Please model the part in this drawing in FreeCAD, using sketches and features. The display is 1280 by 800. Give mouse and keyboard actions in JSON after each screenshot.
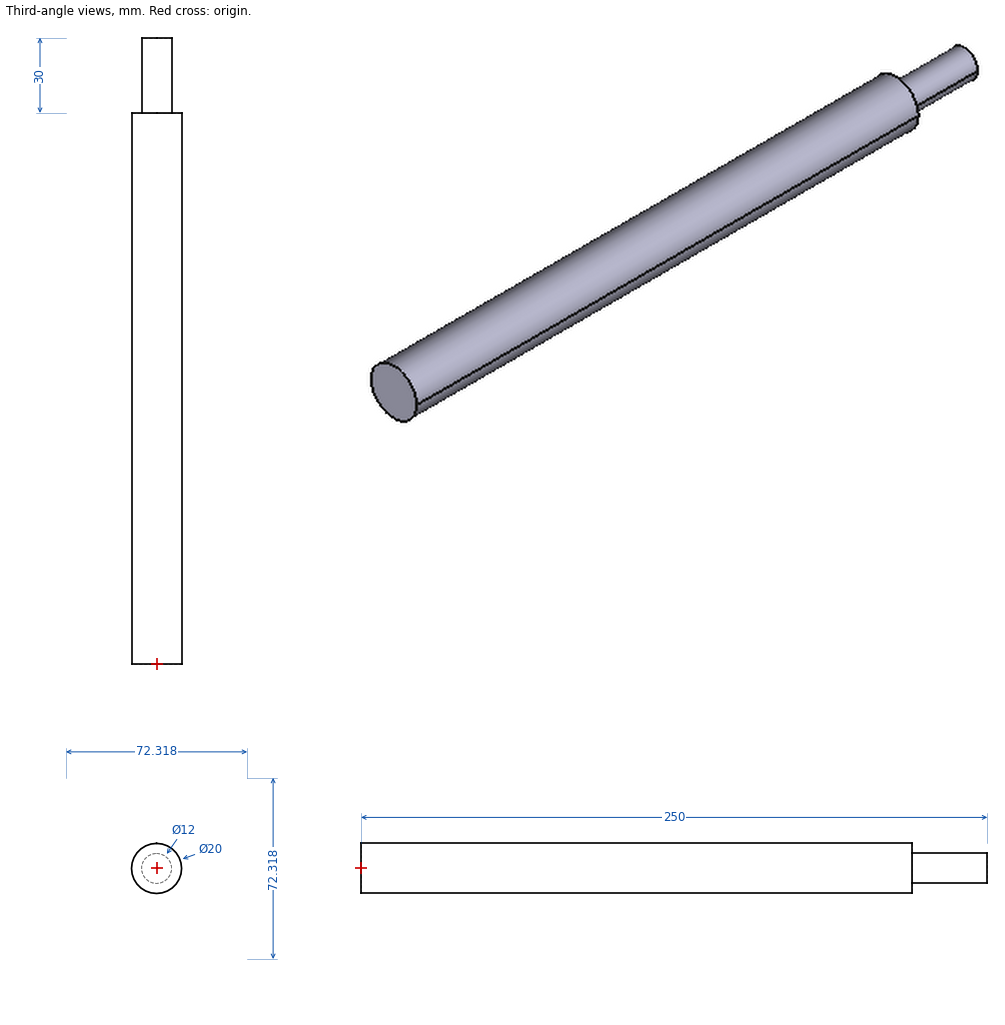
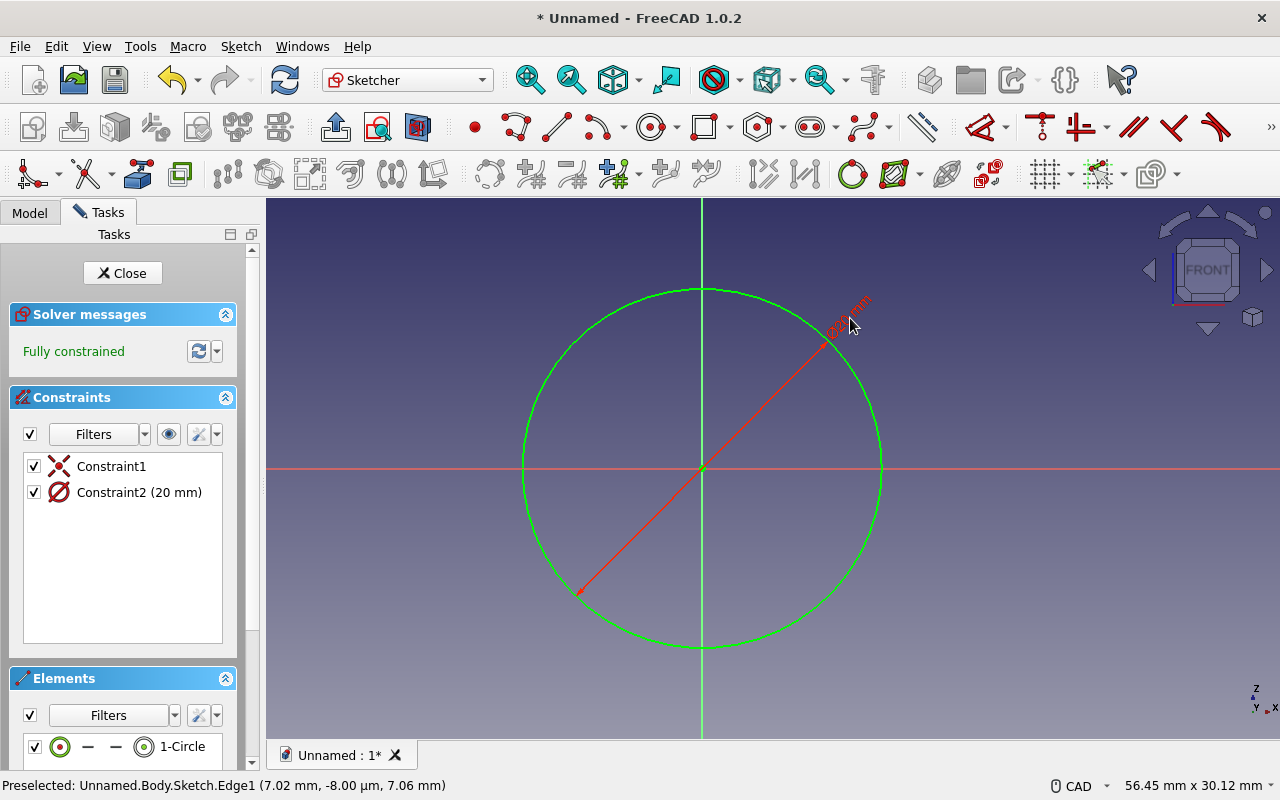
{"action": "left_click", "coordinate": [123, 273]}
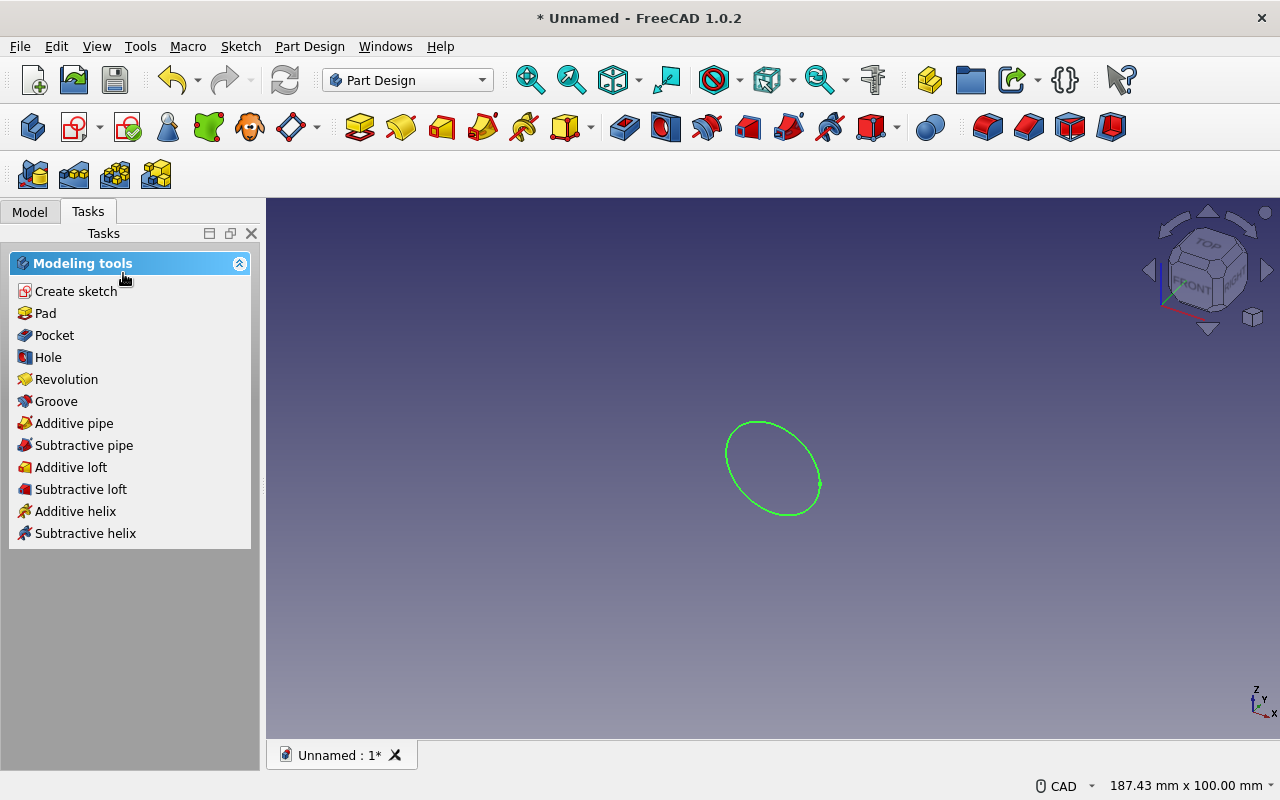
{"action": "left_click", "coordinate": [360, 128]}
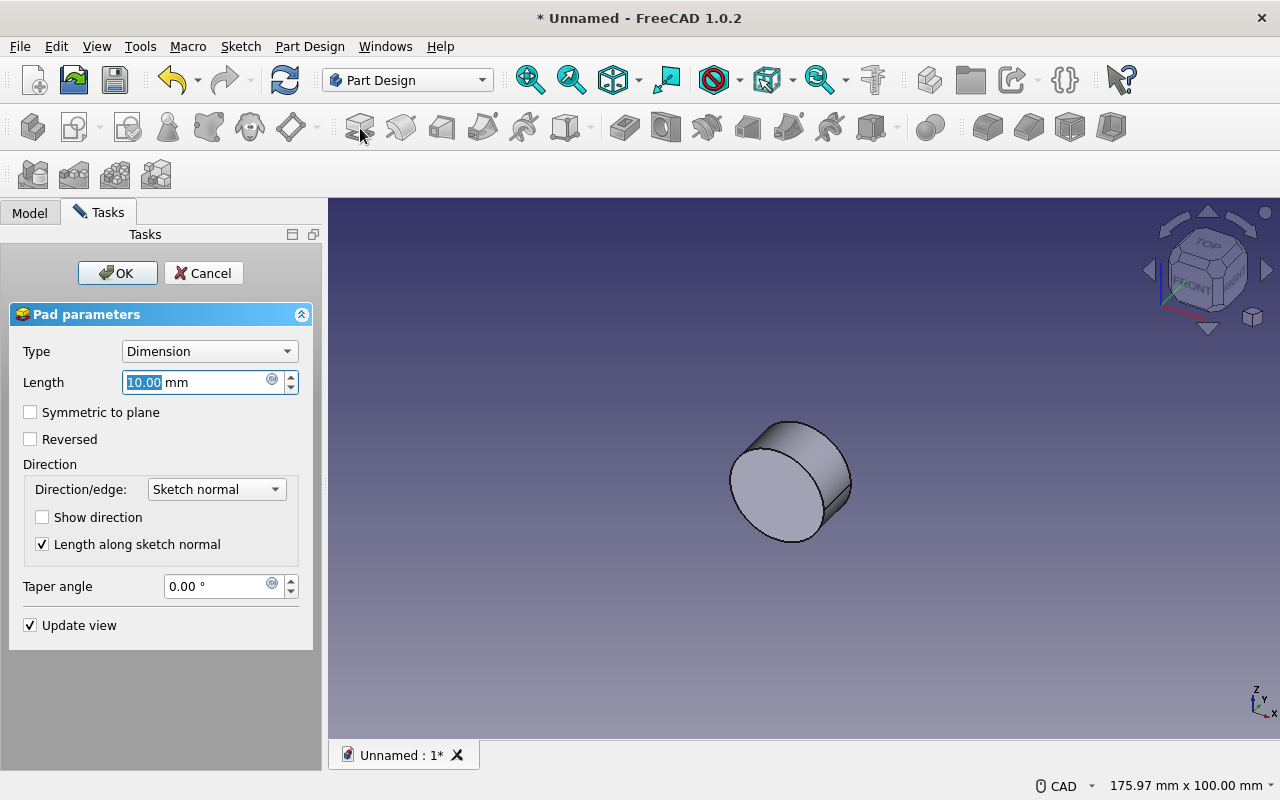
{"action": "type", "text": "250"}
{"action": "key", "text": "Tab"}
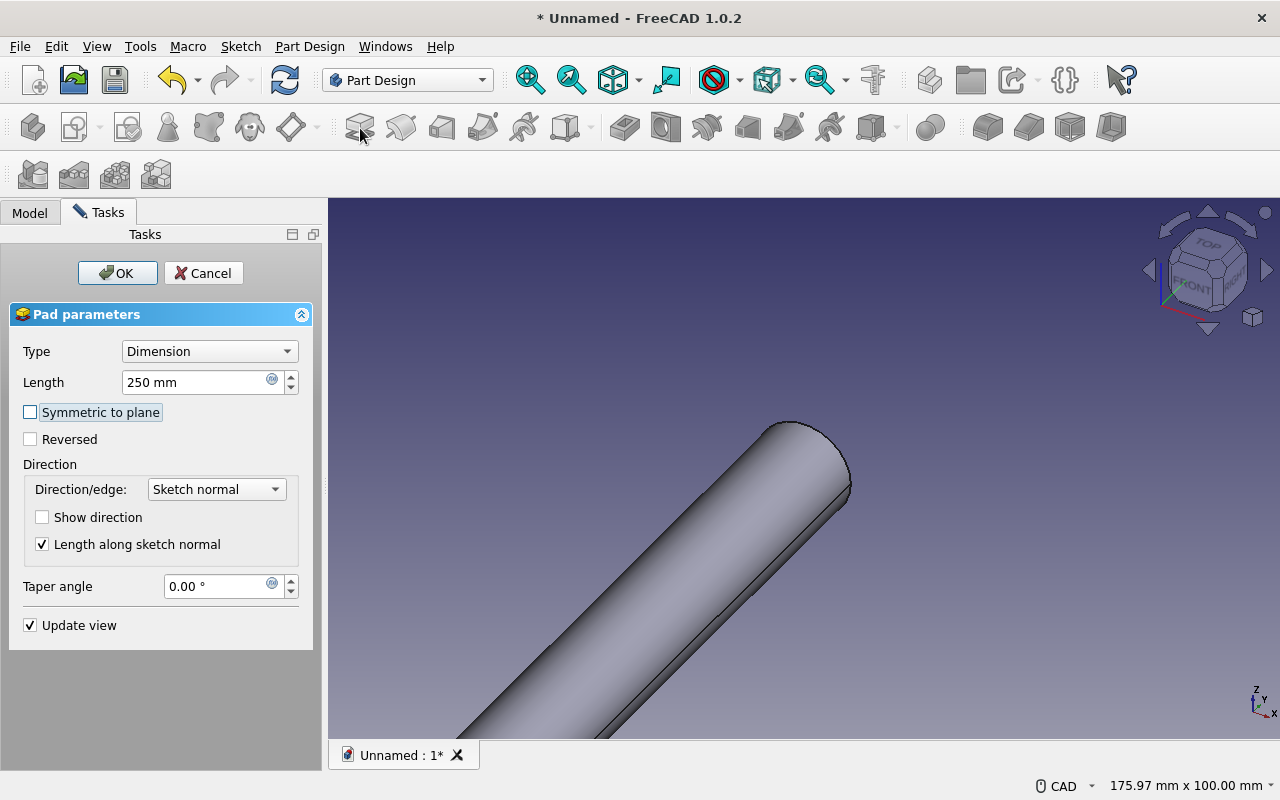
{"action": "left_click", "coordinate": [31, 439]}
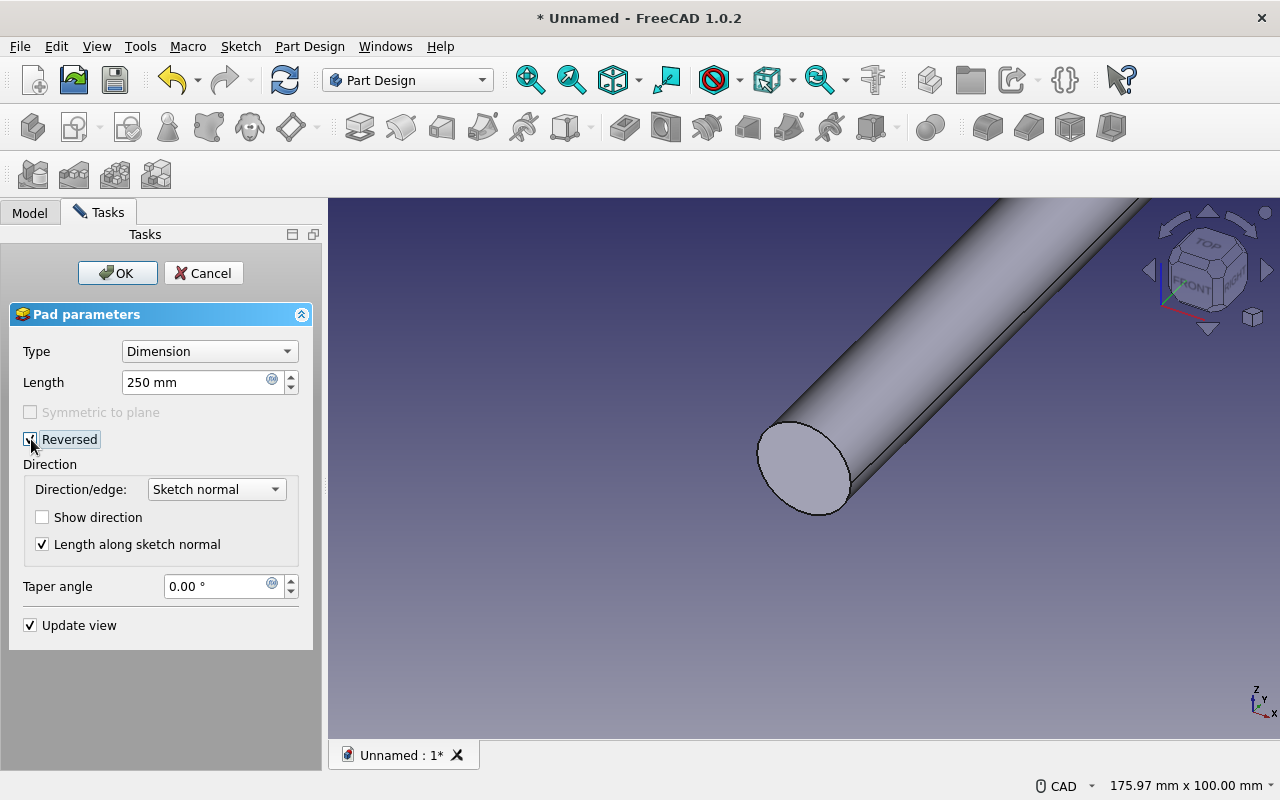
{"action": "left_click", "coordinate": [118, 273]}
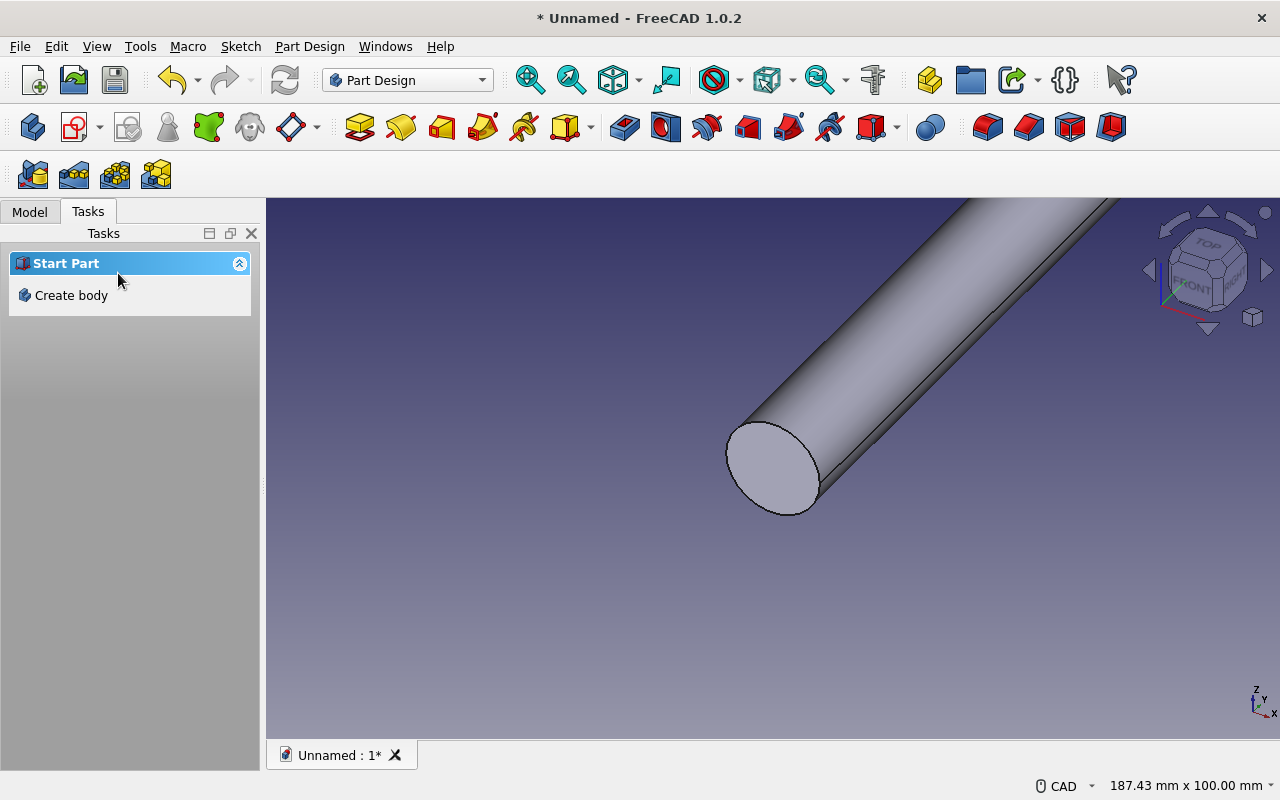
{"action": "left_click", "coordinate": [531, 80]}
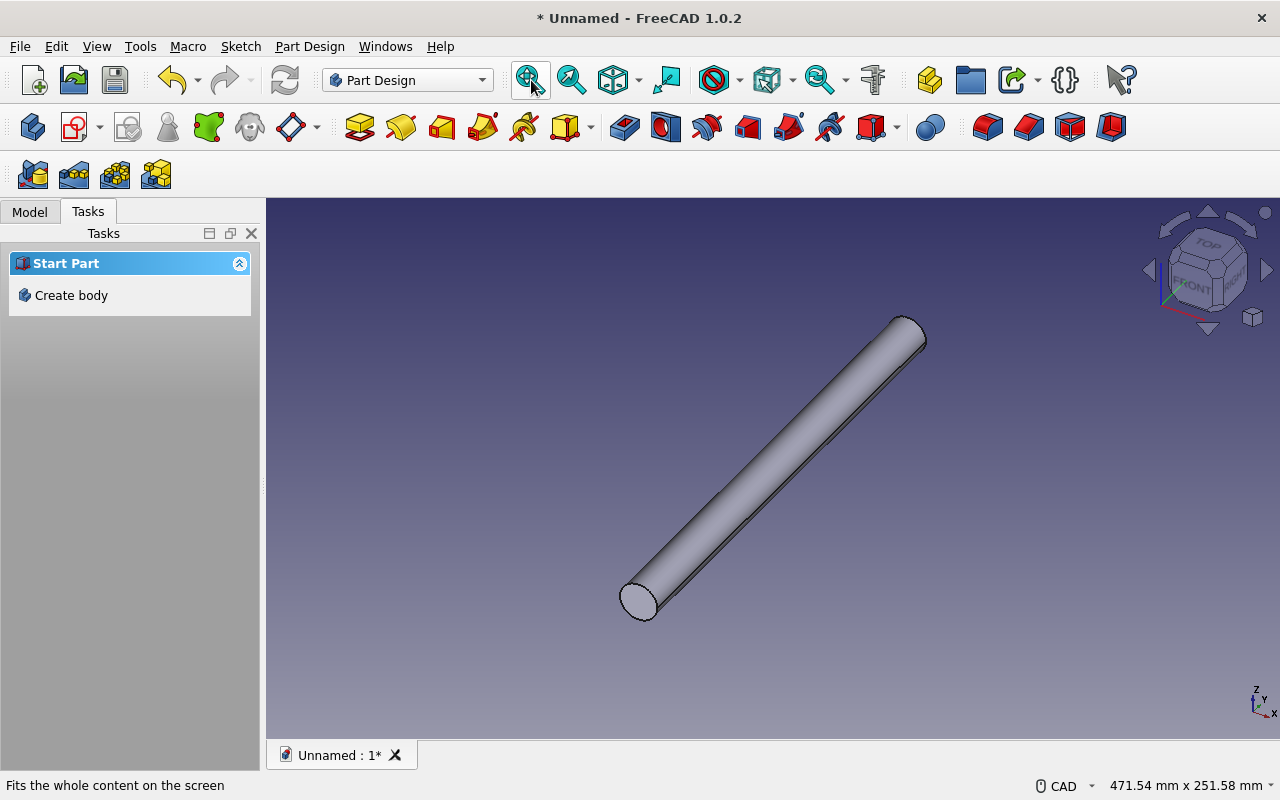
{"action": "key", "text": "4"}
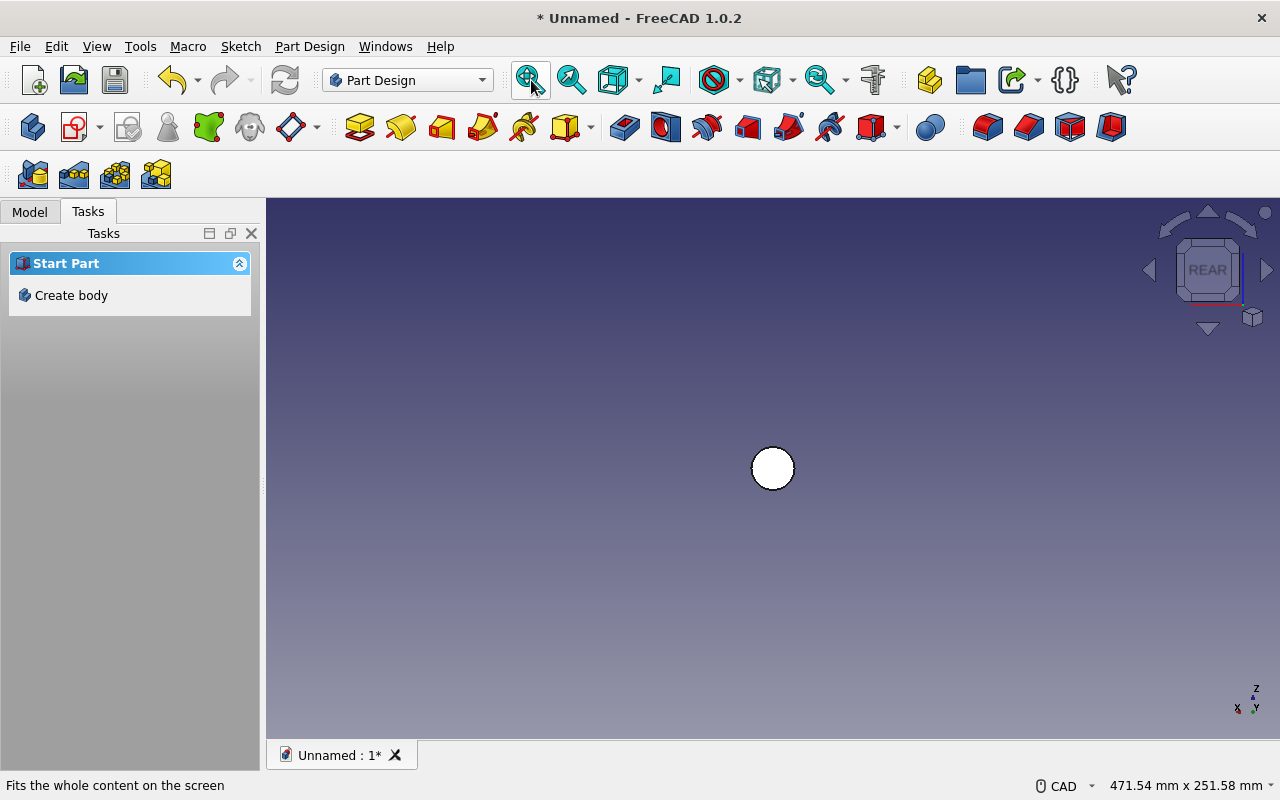
{"action": "left_click", "coordinate": [531, 80]}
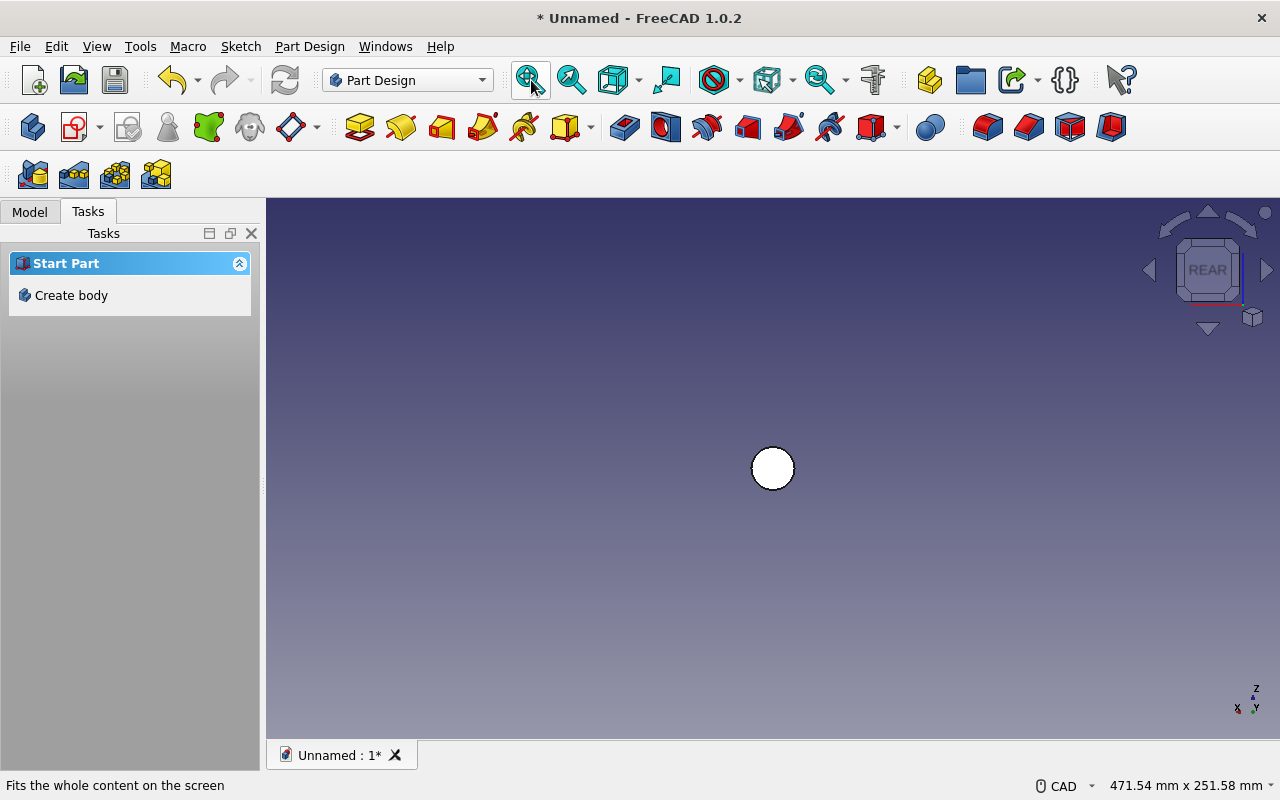
{"action": "left_click", "coordinate": [773, 468]}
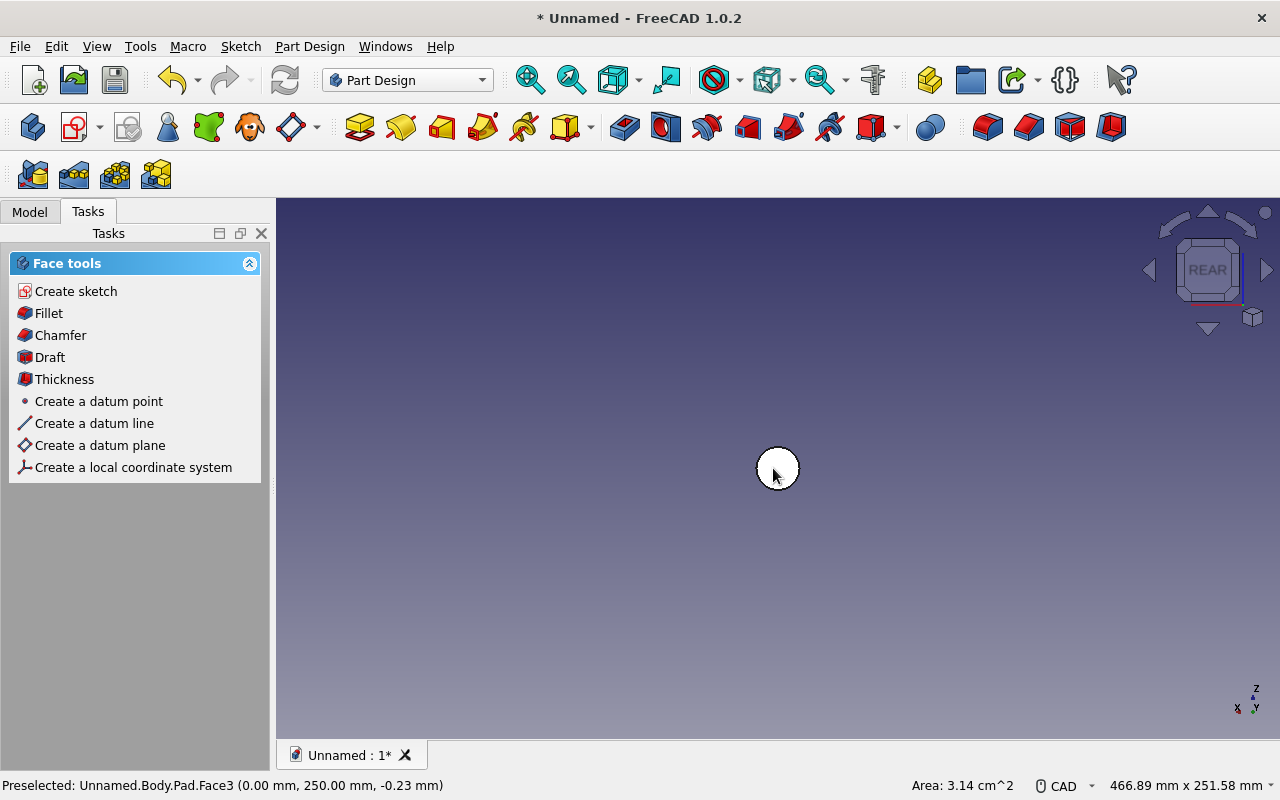
{"action": "left_click", "coordinate": [74, 128]}